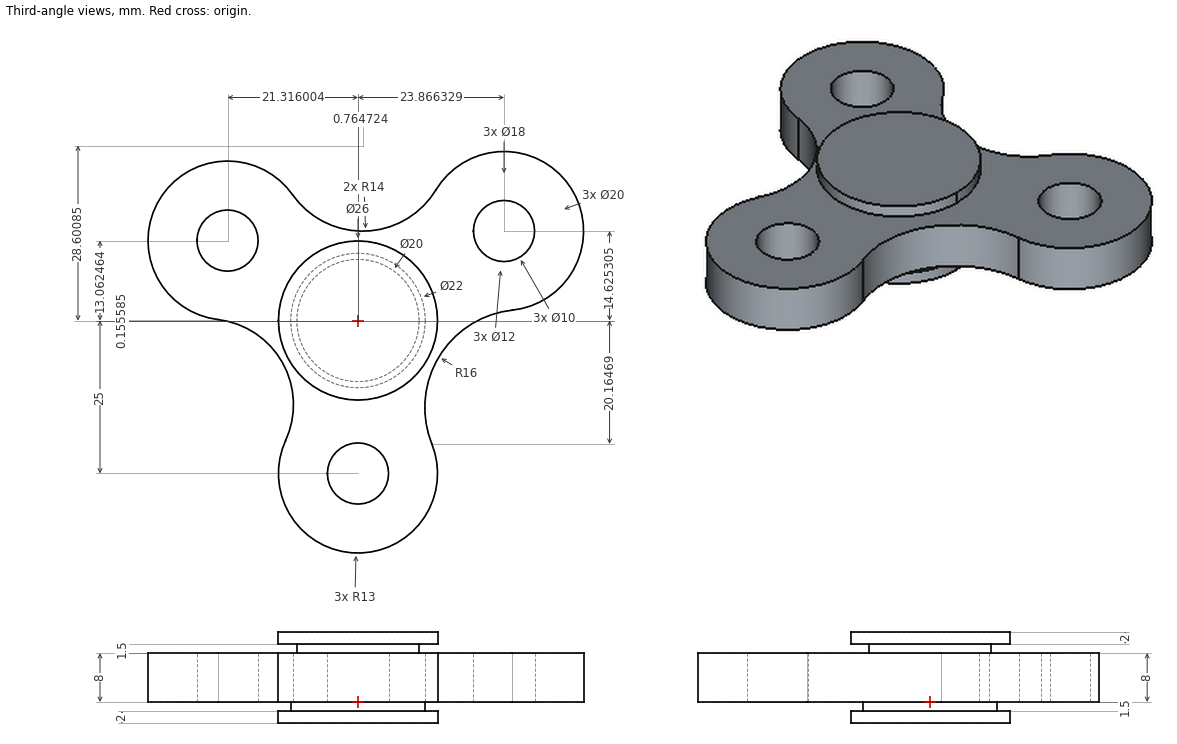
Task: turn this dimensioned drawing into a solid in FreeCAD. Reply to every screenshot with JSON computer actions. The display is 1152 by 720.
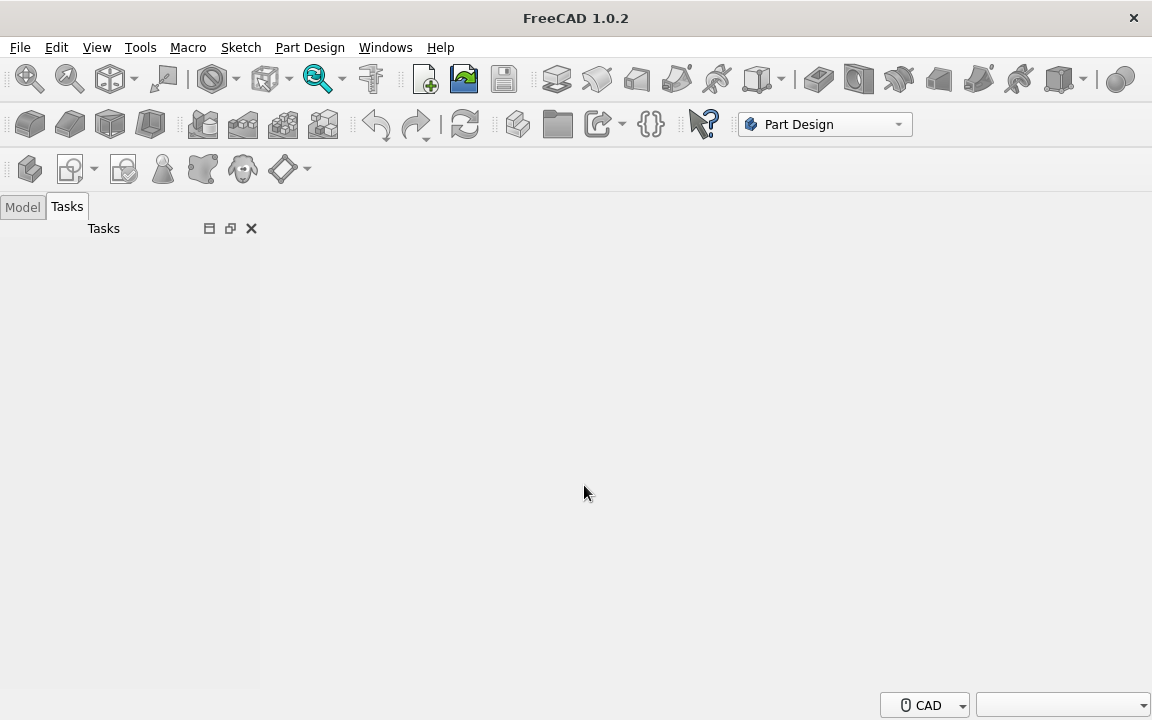
{"action": "left_click", "coordinate": [424, 80]}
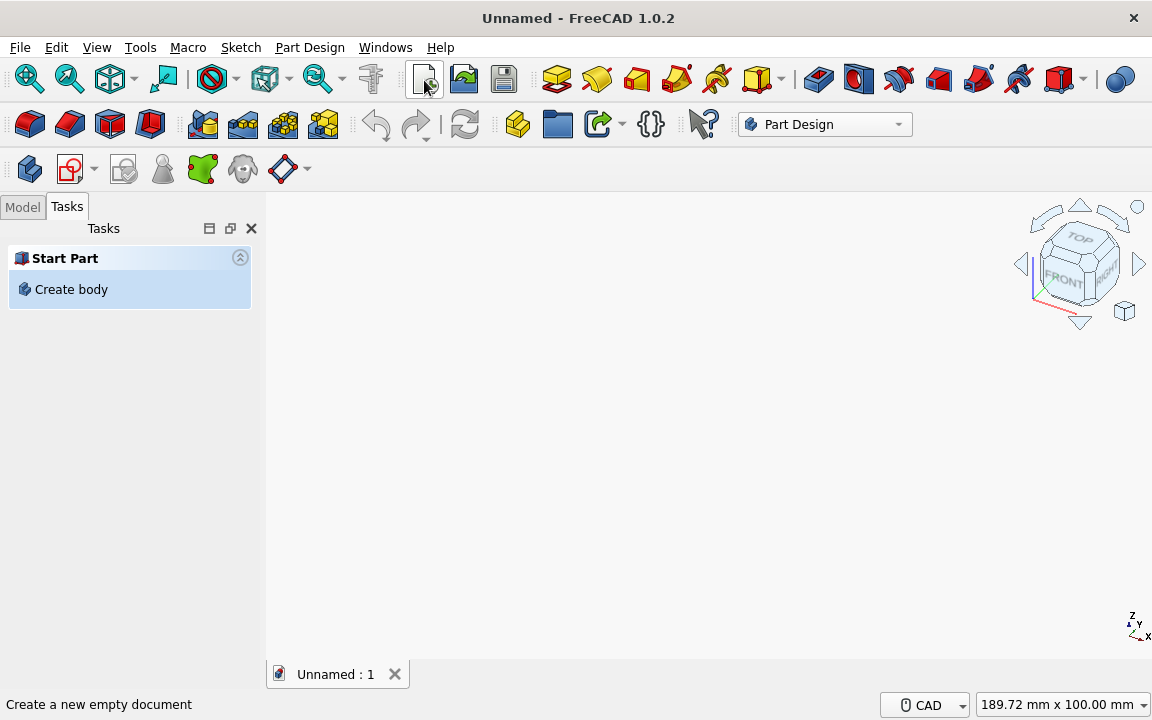
{"action": "left_click", "coordinate": [70, 170]}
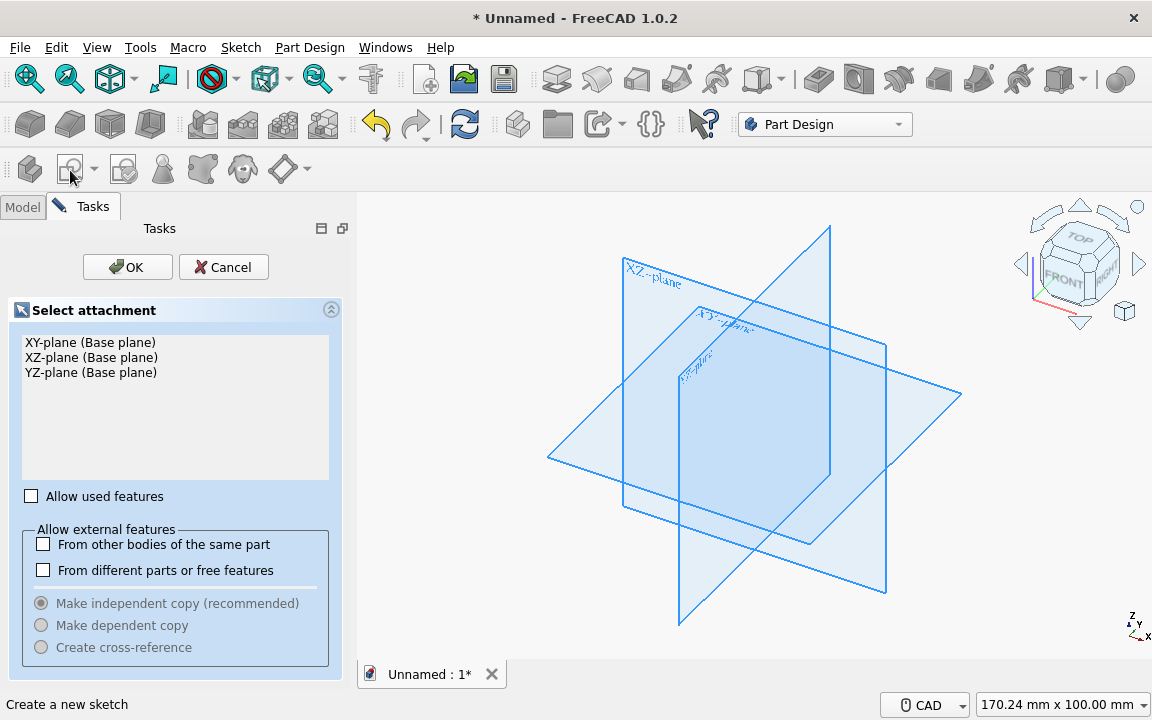
{"action": "left_click", "coordinate": [82, 342]}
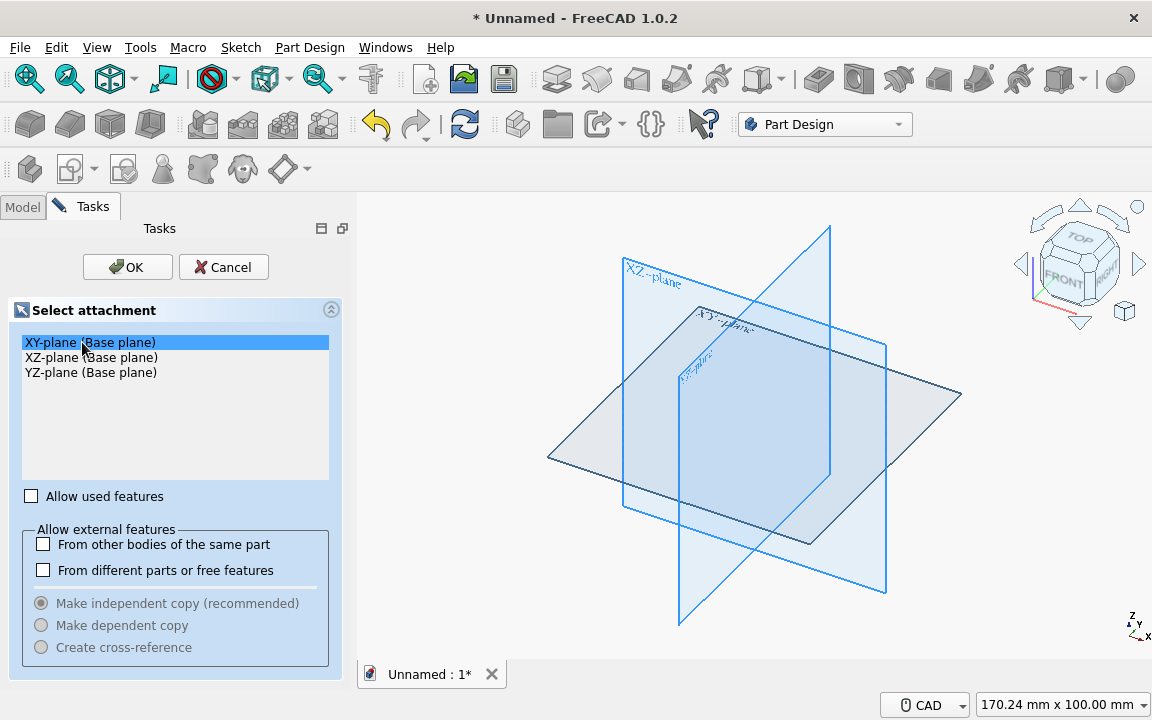
{"action": "left_click", "coordinate": [128, 267]}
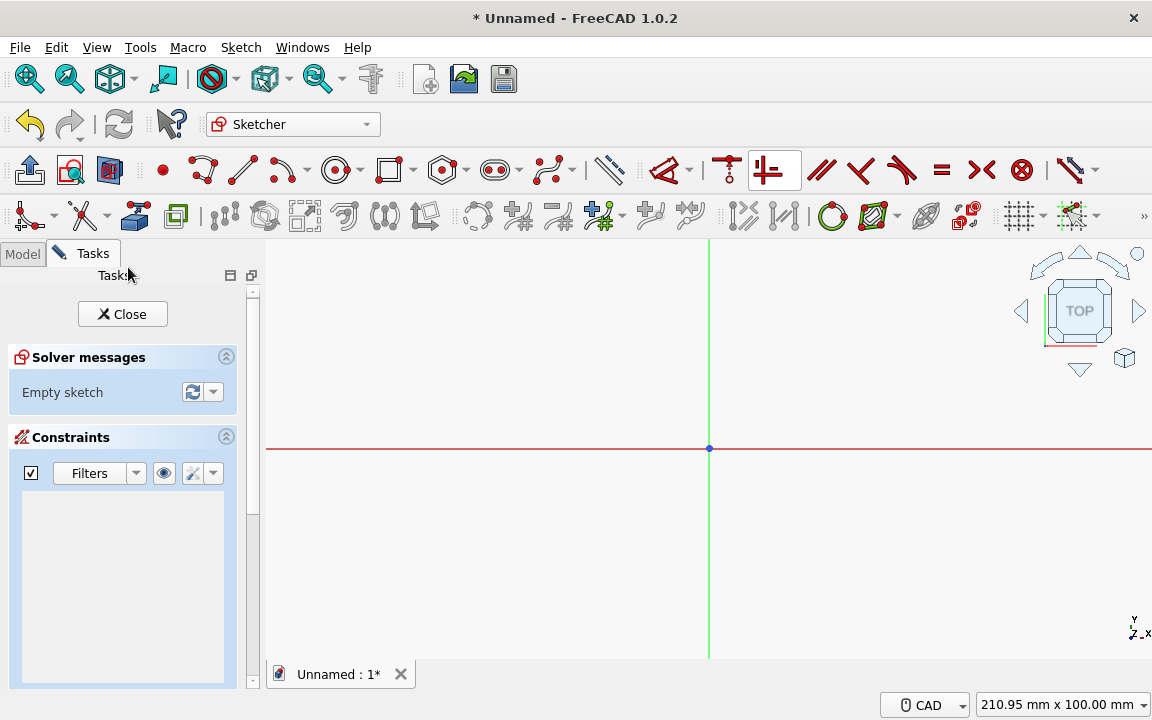
{"action": "scroll", "coordinate": [309, 293], "scroll_direction": "down", "scroll_amount": 1}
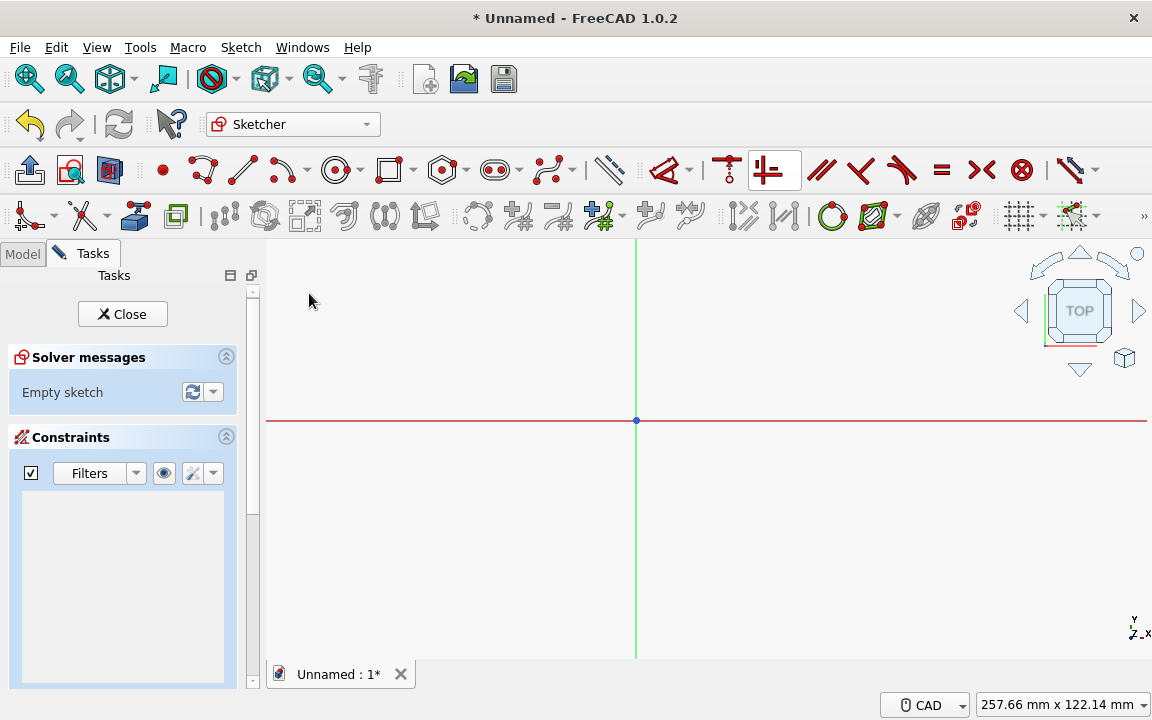
{"action": "left_click", "coordinate": [310, 170]}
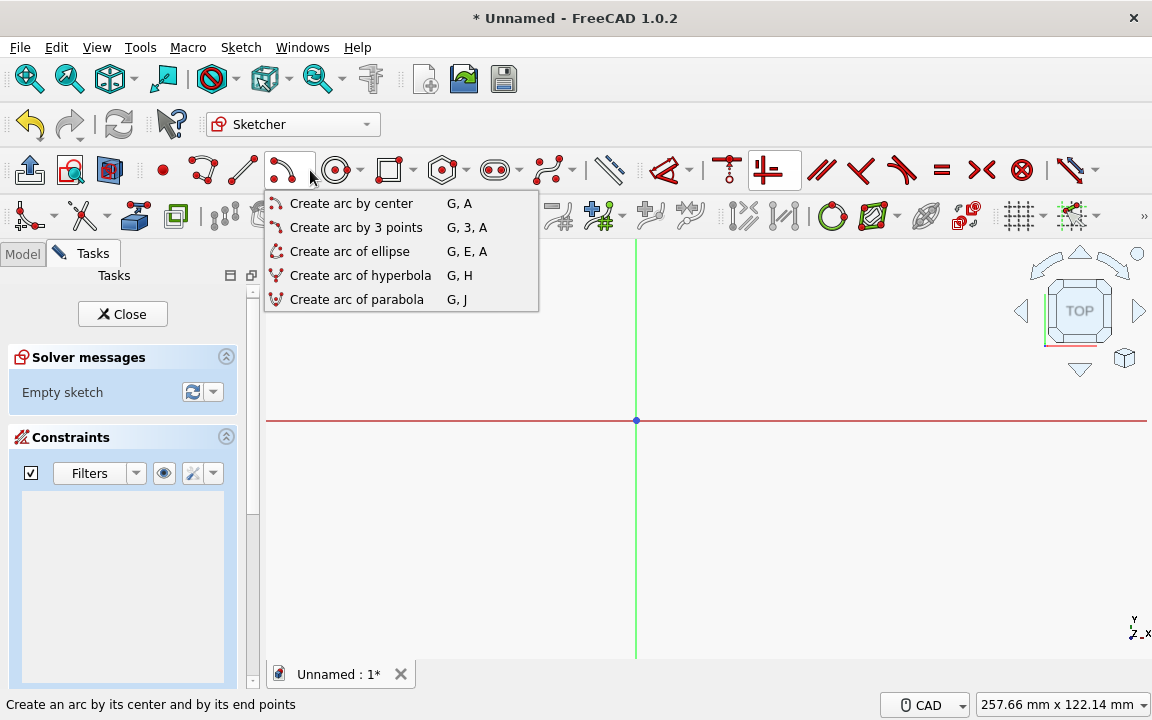
{"action": "left_click", "coordinate": [402, 227]}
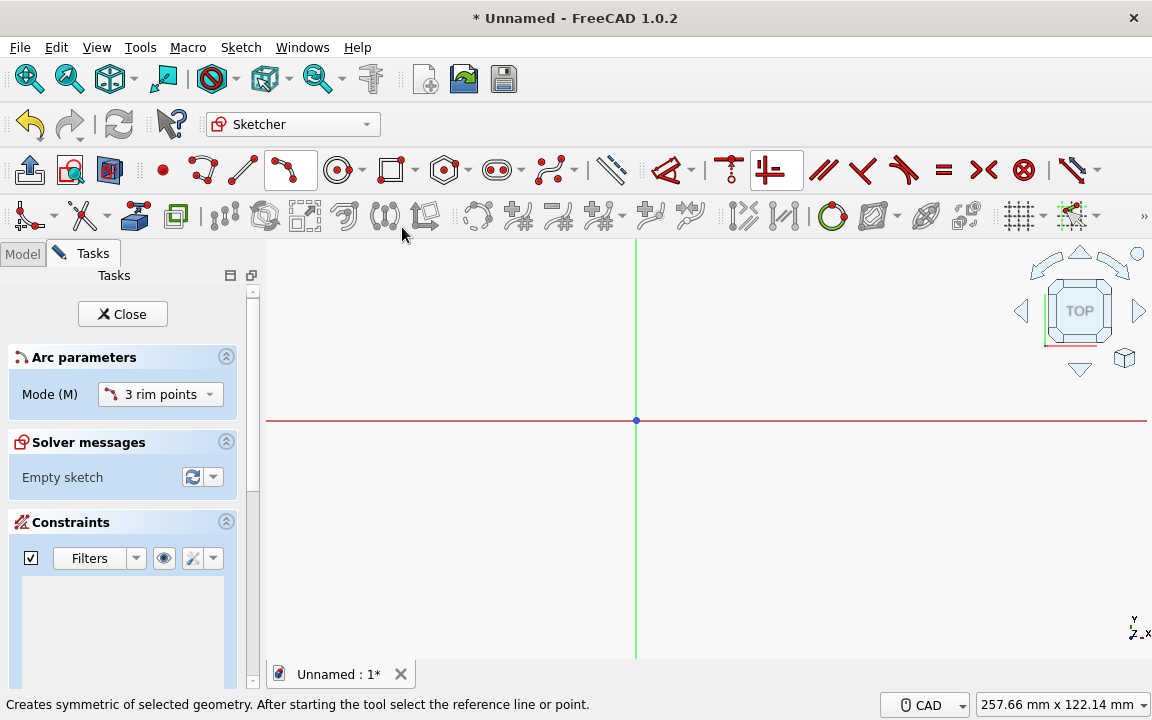
{"action": "scroll", "coordinate": [558, 420], "scroll_direction": "up", "scroll_amount": 17}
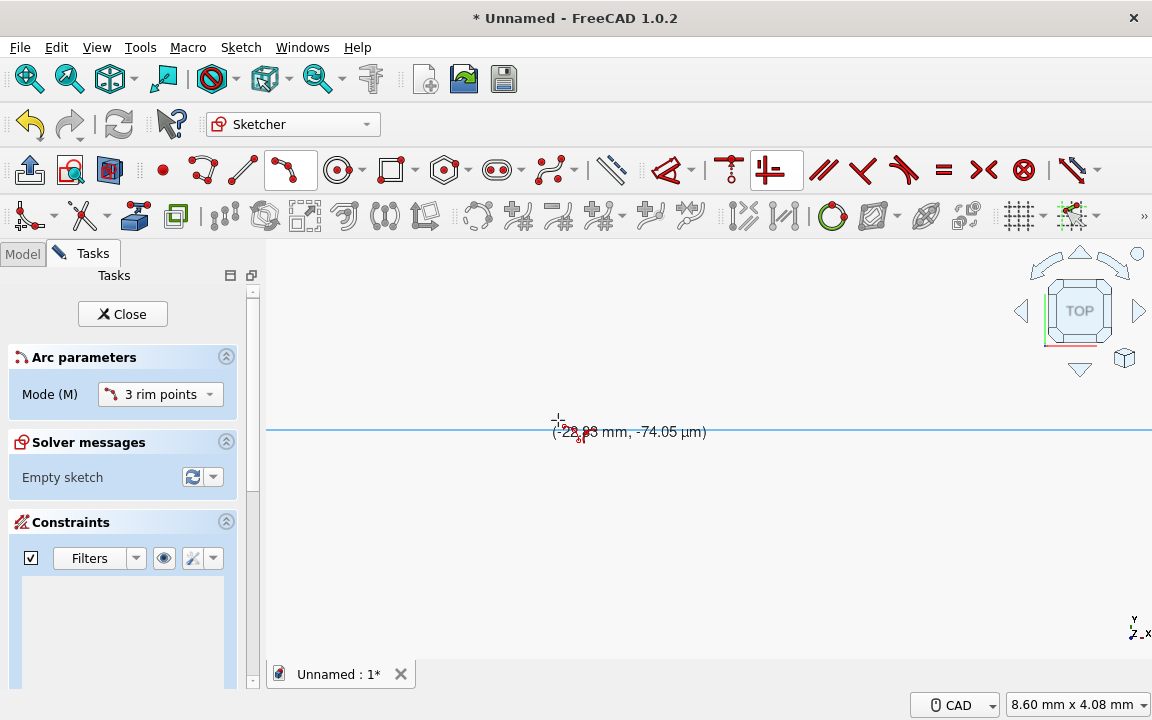
{"action": "left_click", "coordinate": [544, 414]}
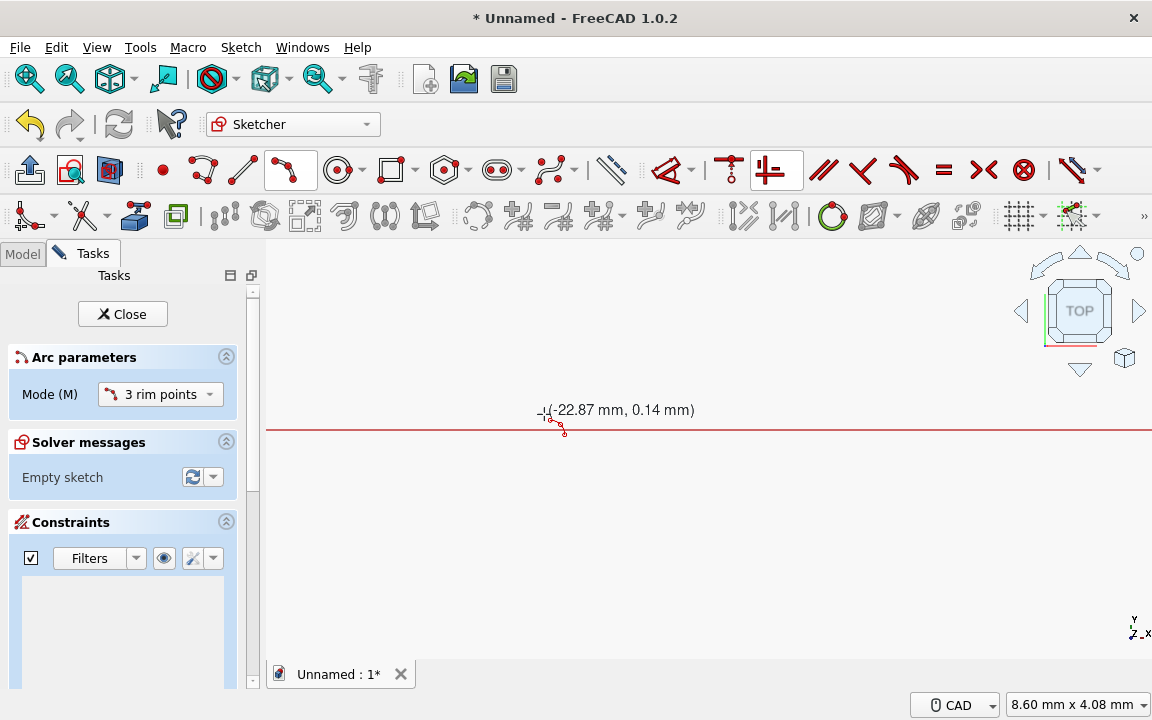
{"action": "scroll", "coordinate": [516, 406], "scroll_direction": "down", "scroll_amount": 15}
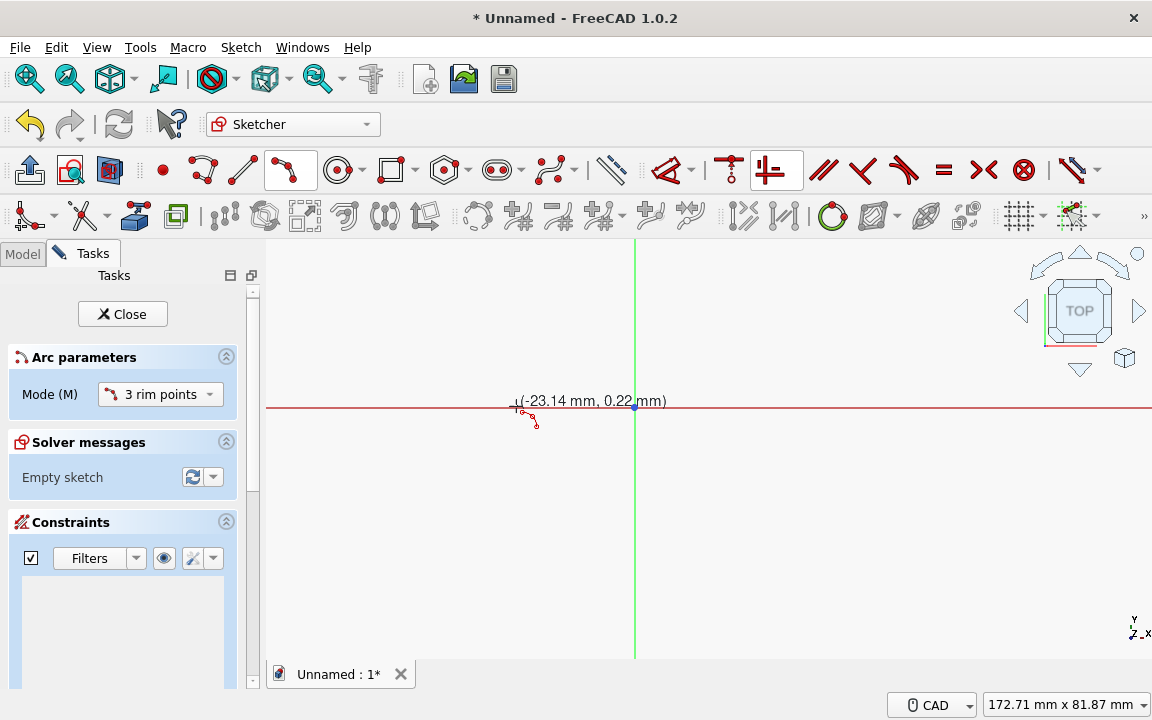
{"action": "left_click", "coordinate": [574, 508]}
{"action": "left_click", "coordinate": [572, 443]}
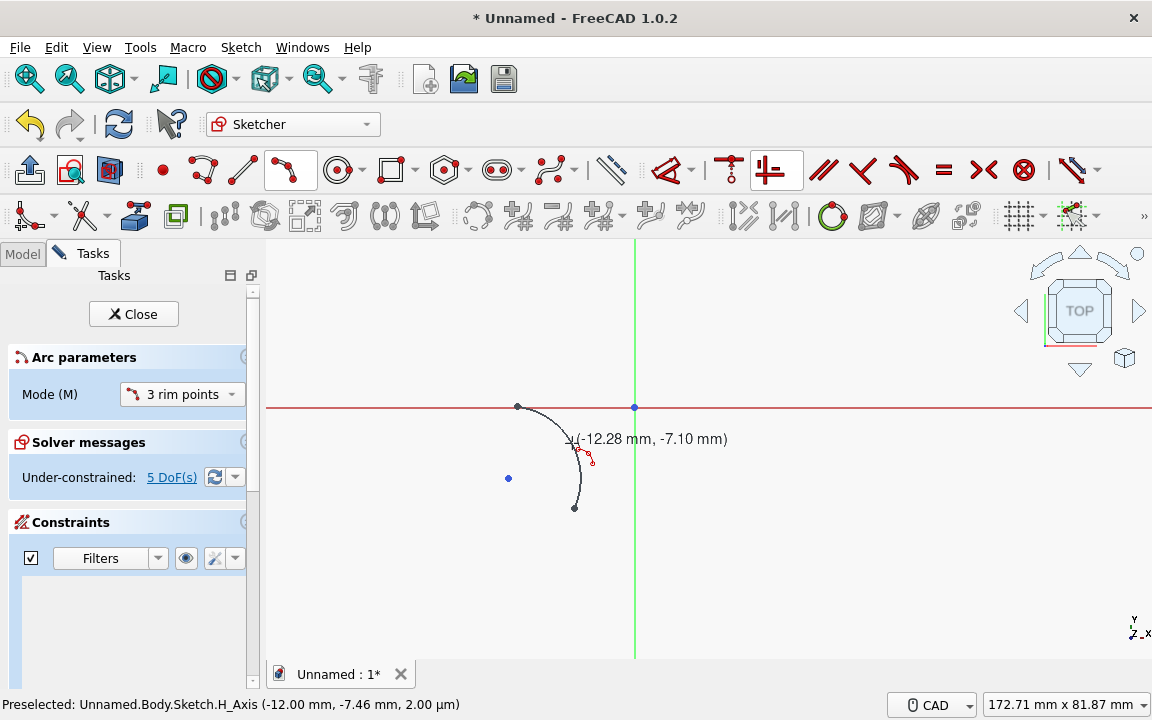
{"action": "left_click", "coordinate": [574, 509]}
{"action": "left_click", "coordinate": [697, 511]}
{"action": "left_click", "coordinate": [608, 597]}